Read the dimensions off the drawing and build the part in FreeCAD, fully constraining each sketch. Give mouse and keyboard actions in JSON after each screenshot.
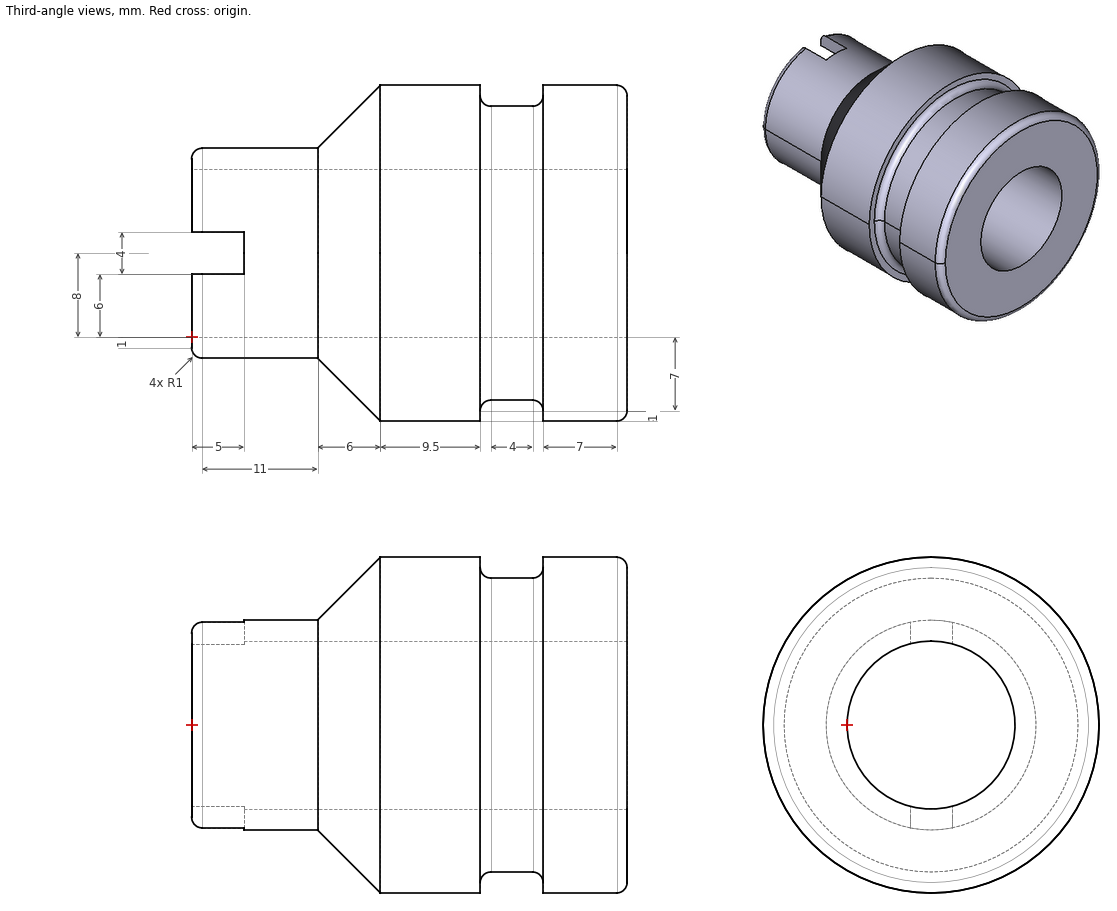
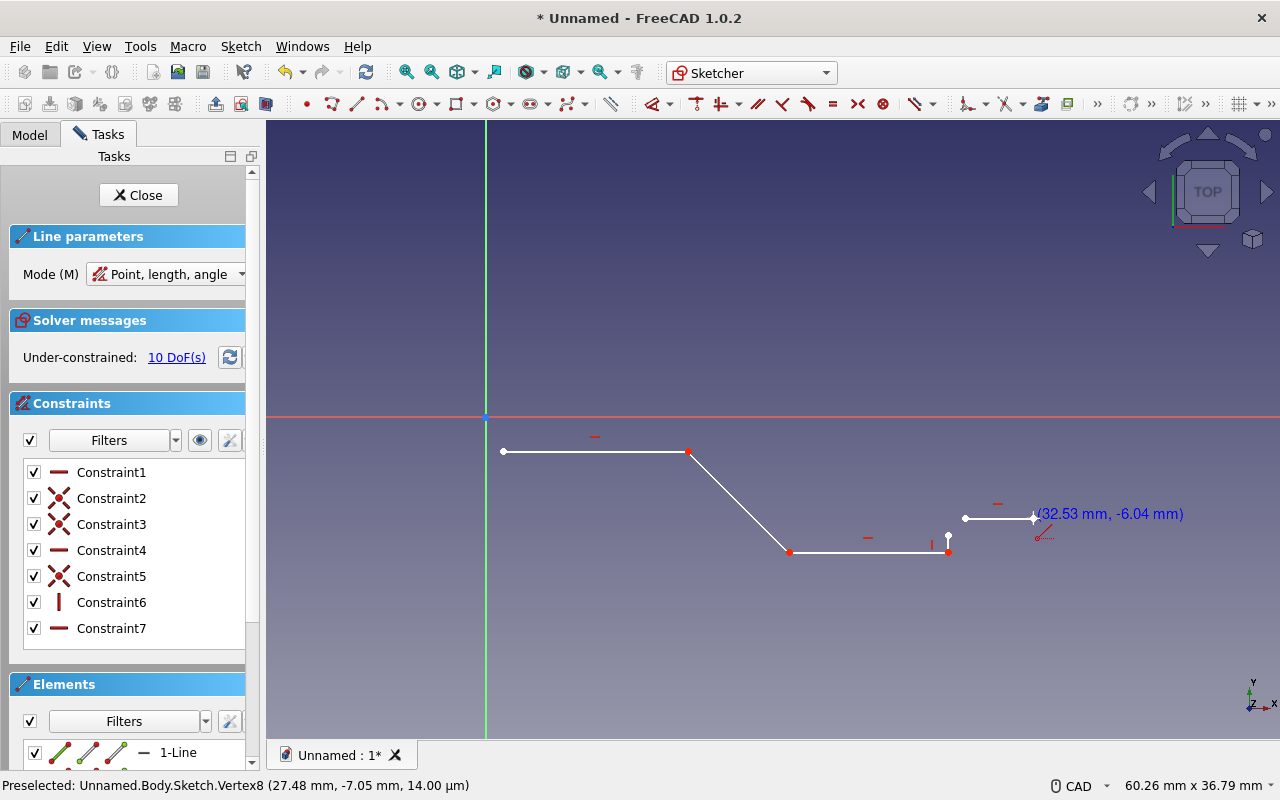
{"action": "key", "text": "g m"}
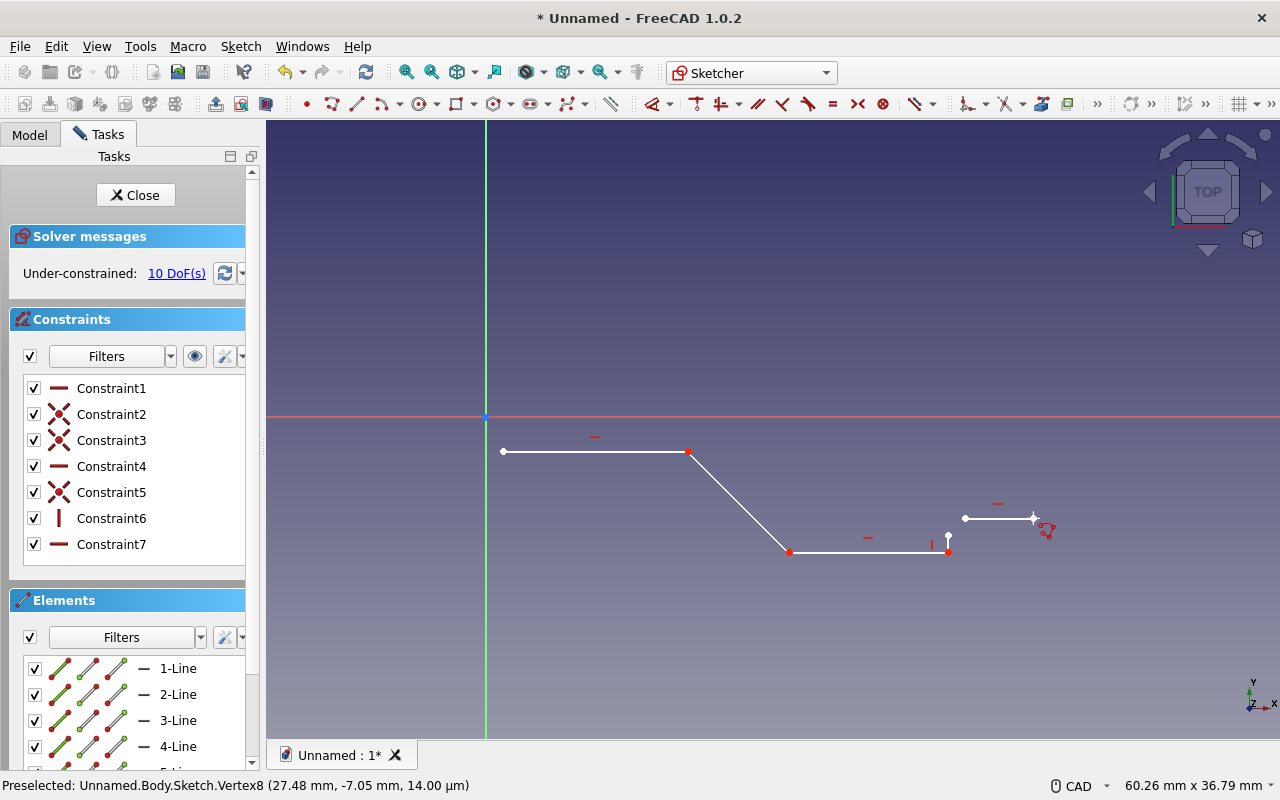
{"action": "left_click", "coordinate": [1049, 535]}
{"action": "left_click", "coordinate": [1049, 552]}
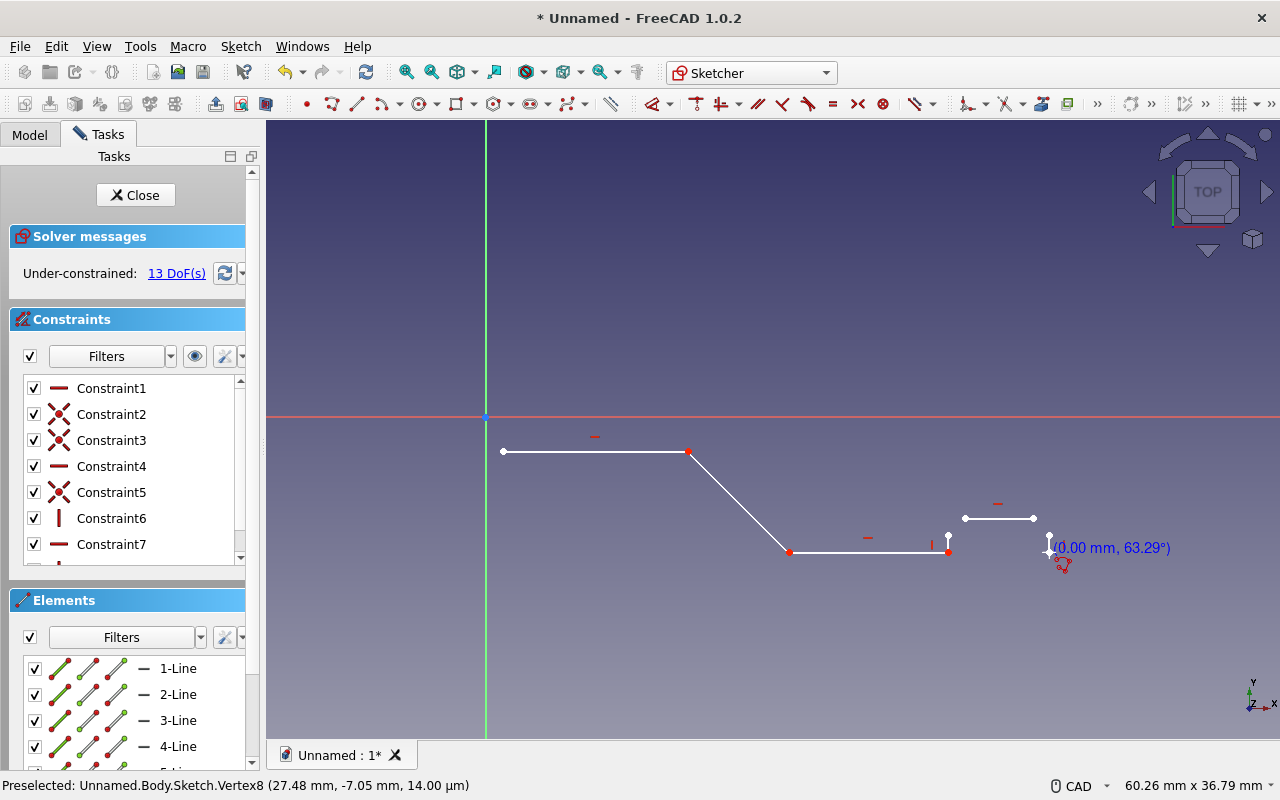
{"action": "scroll", "coordinate": [439, 454], "scroll_direction": "down", "scroll_amount": 2}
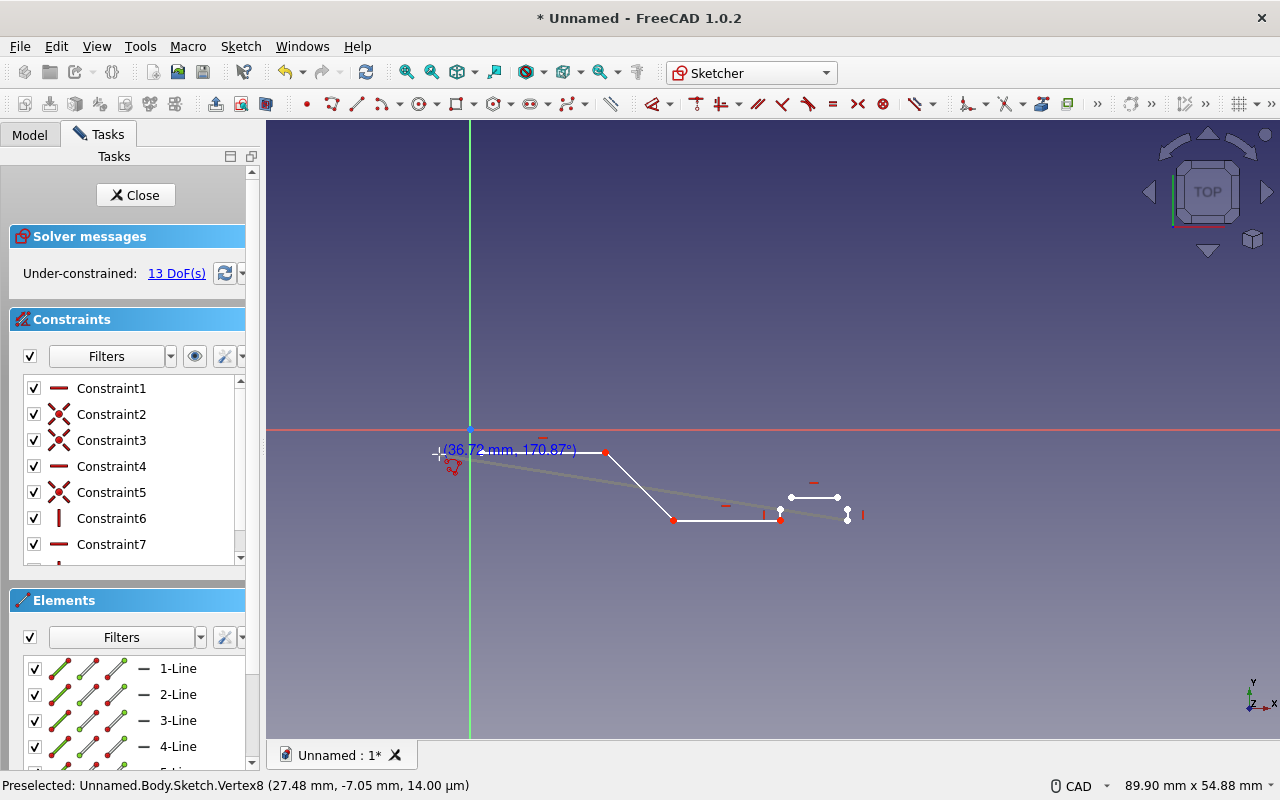
{"action": "left_click", "coordinate": [927, 520]}
{"action": "right_click", "coordinate": [927, 520]}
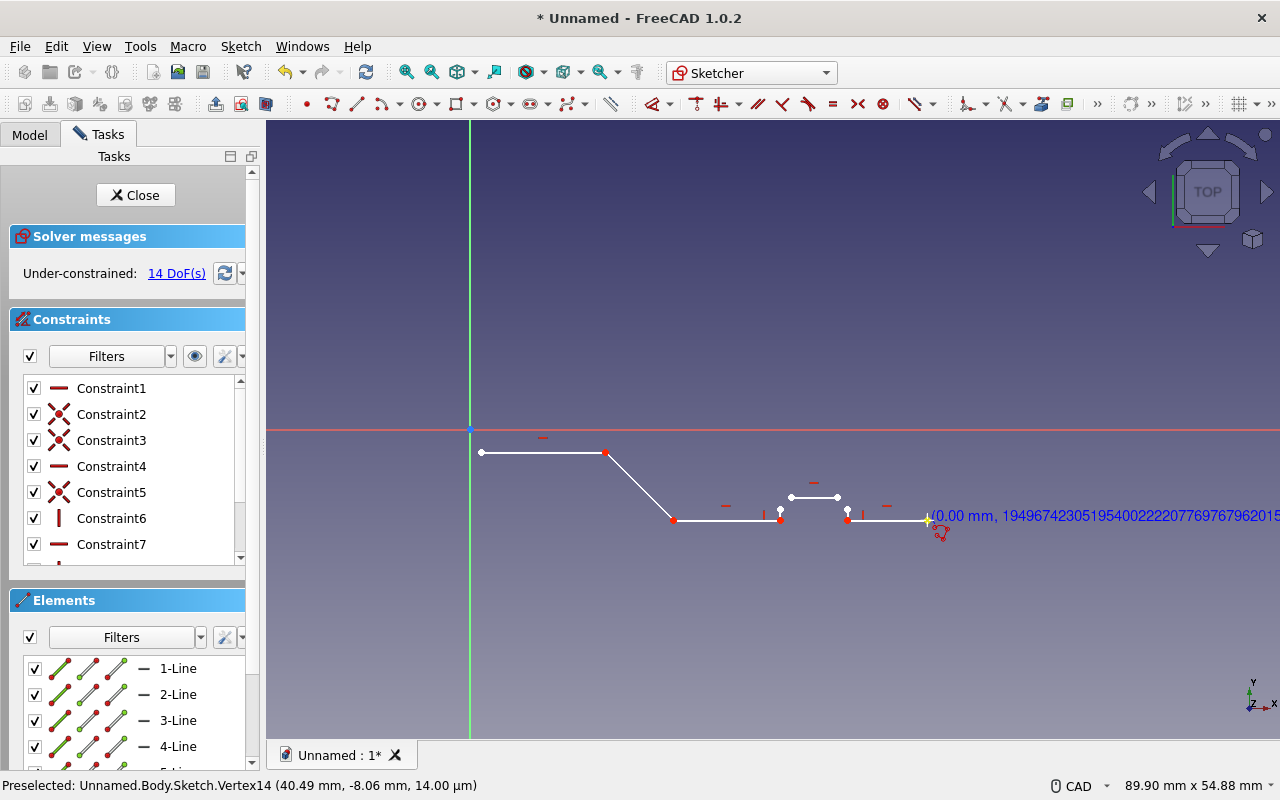
{"action": "left_click", "coordinate": [938, 509]}
{"action": "left_click", "coordinate": [938, 430]}
{"action": "left_click", "coordinate": [470, 430]}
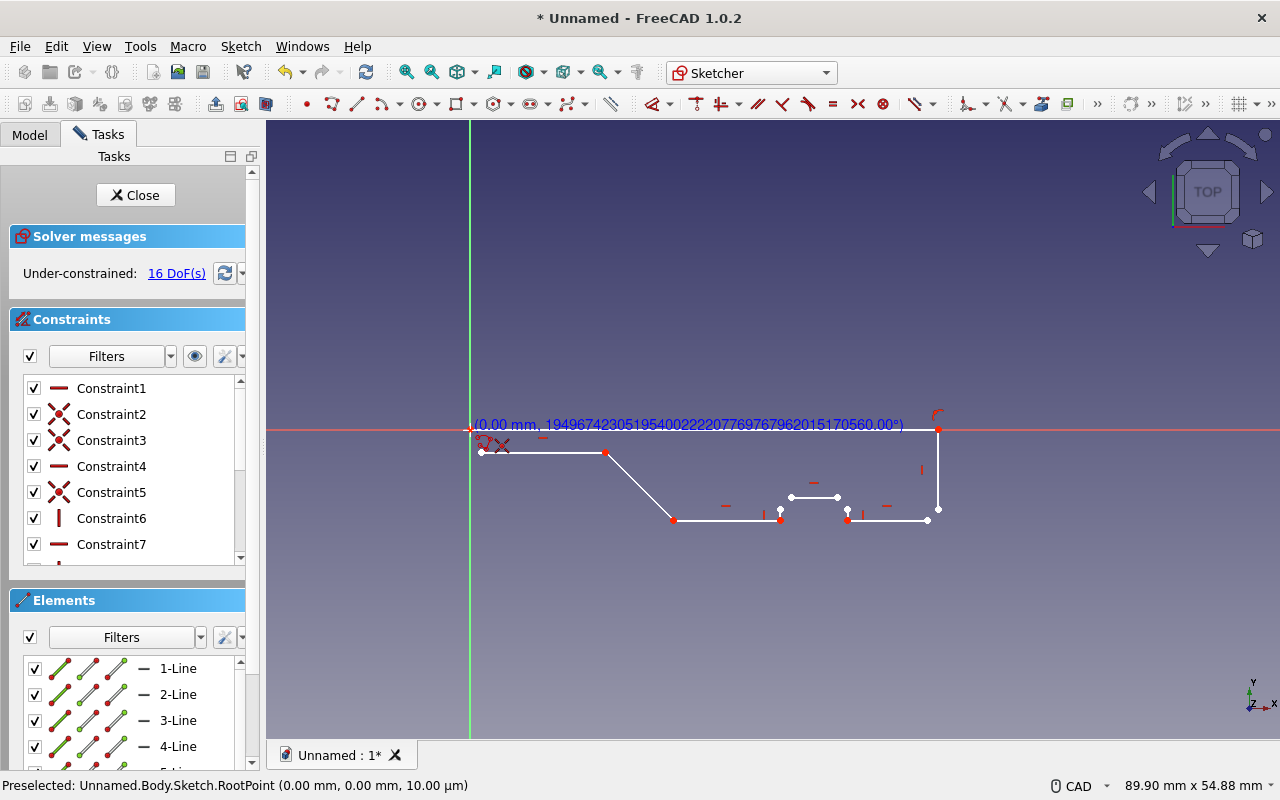
{"action": "scroll", "coordinate": [470, 441], "scroll_direction": "up", "scroll_amount": 2}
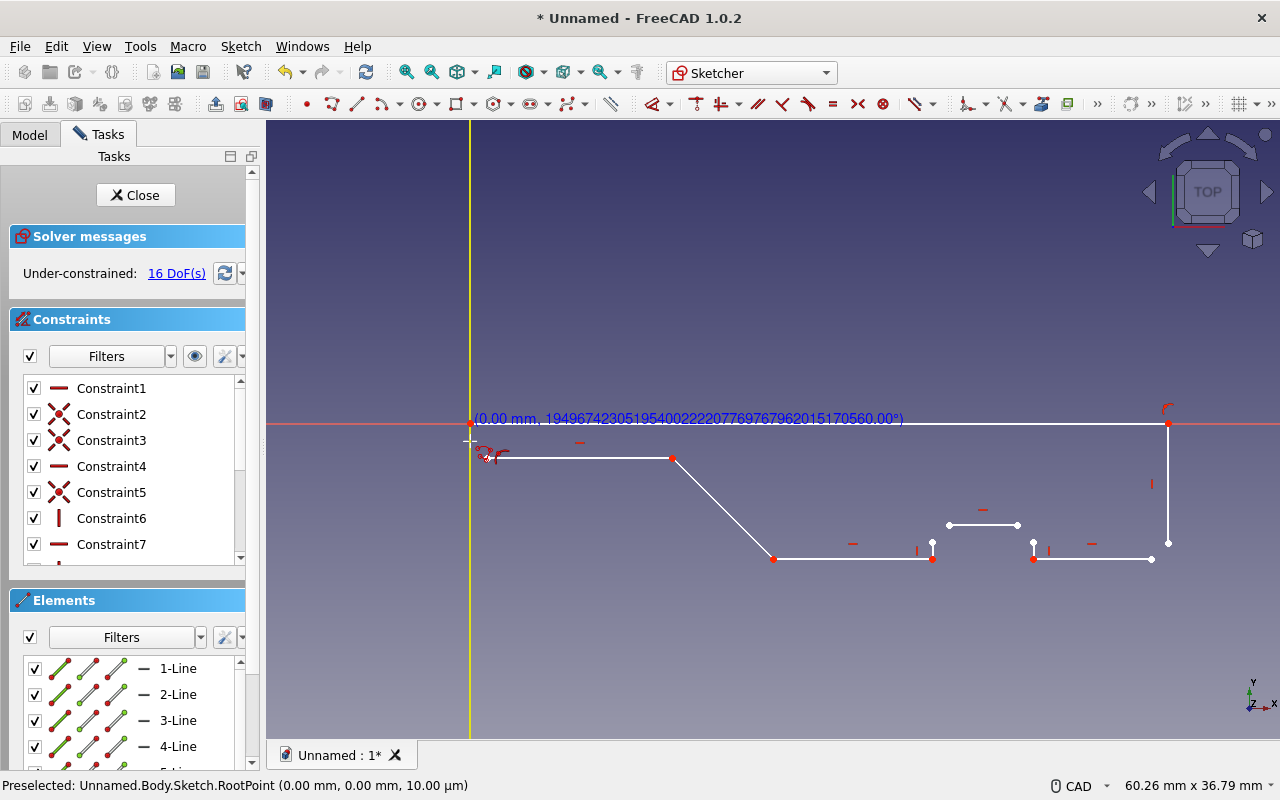
{"action": "left_click", "coordinate": [479, 441]}
{"action": "right_click", "coordinate": [479, 441]}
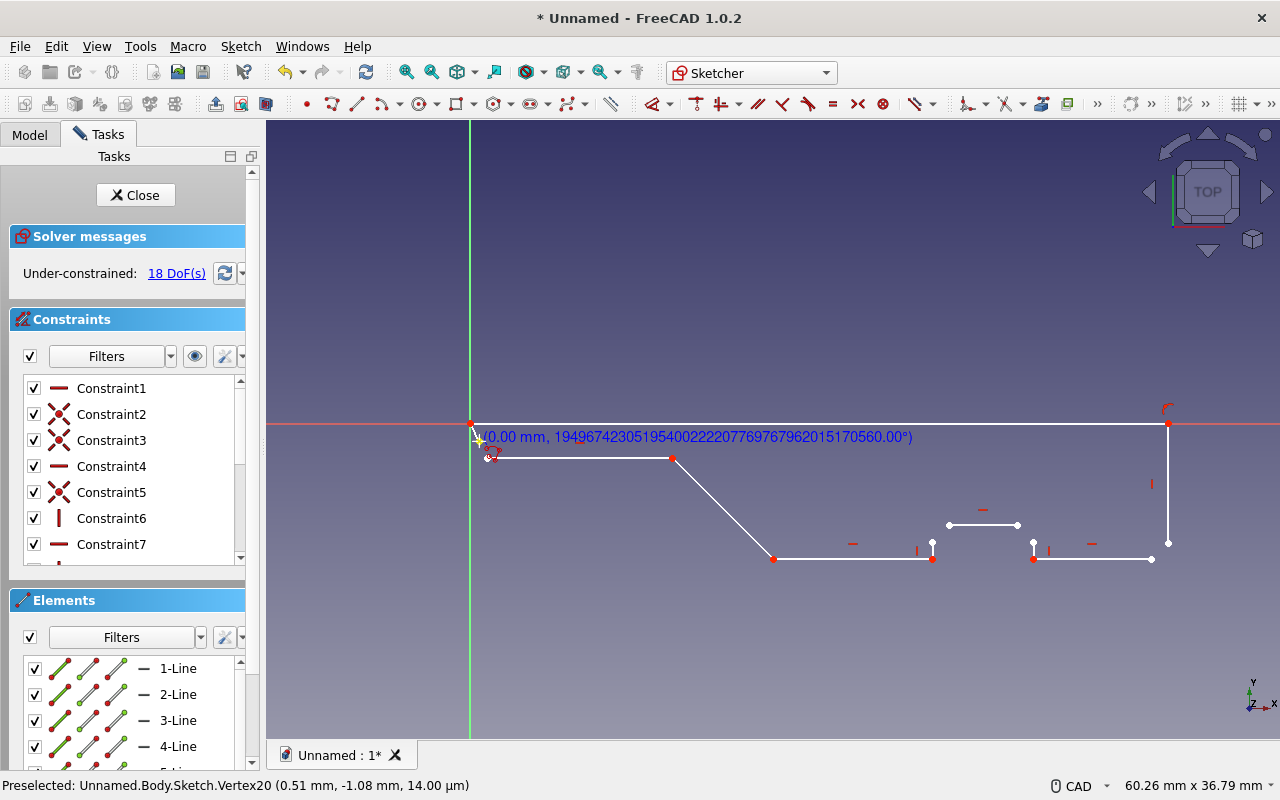
{"action": "key", "text": "g 3 a"}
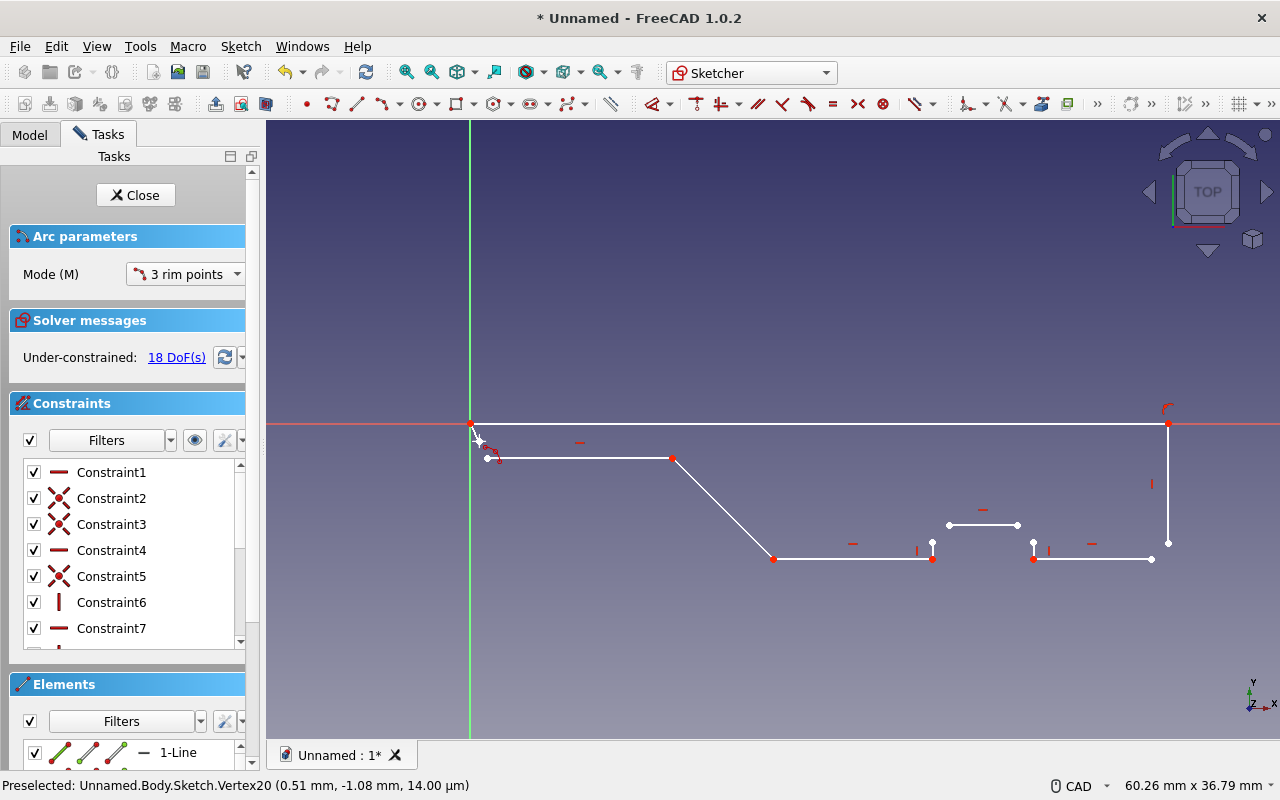
{"action": "scroll", "coordinate": [933, 542], "scroll_direction": "up", "scroll_amount": 4}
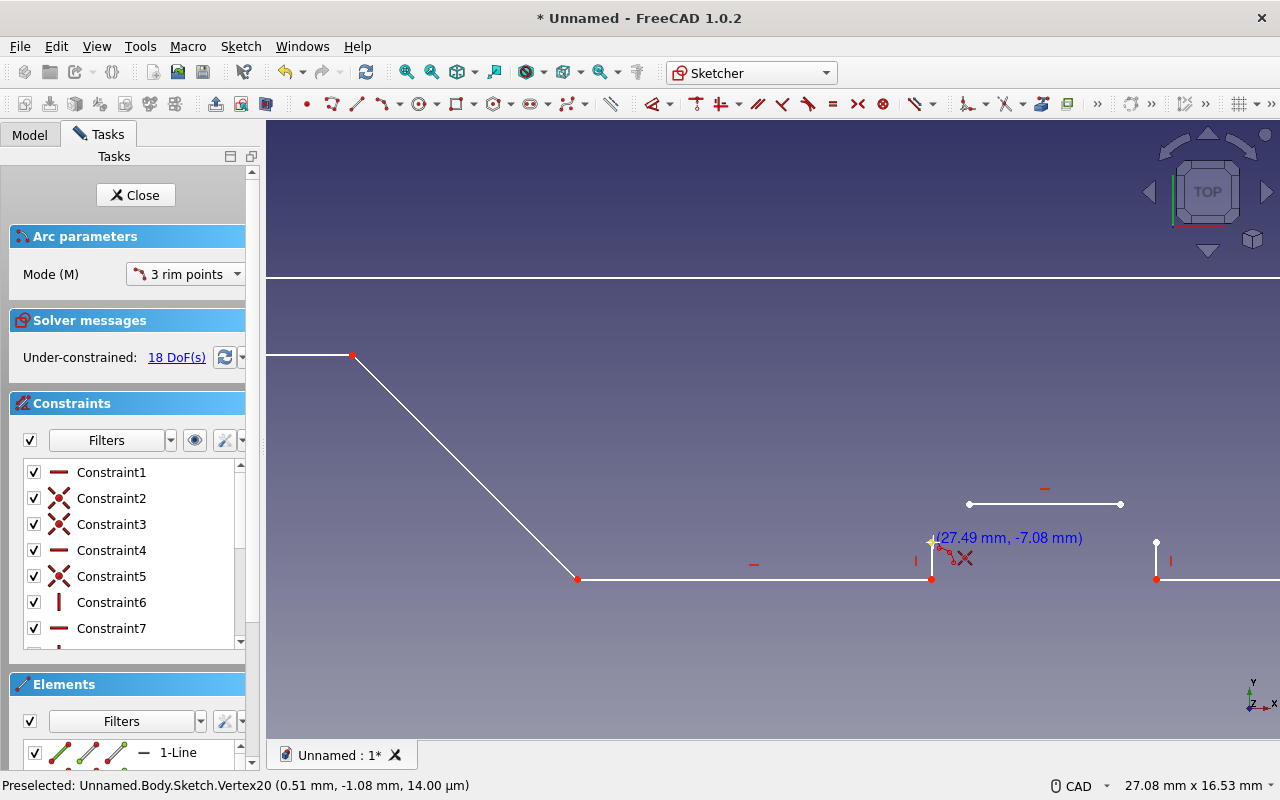
{"action": "left_click", "coordinate": [932, 542]}
{"action": "left_click", "coordinate": [969, 504]}